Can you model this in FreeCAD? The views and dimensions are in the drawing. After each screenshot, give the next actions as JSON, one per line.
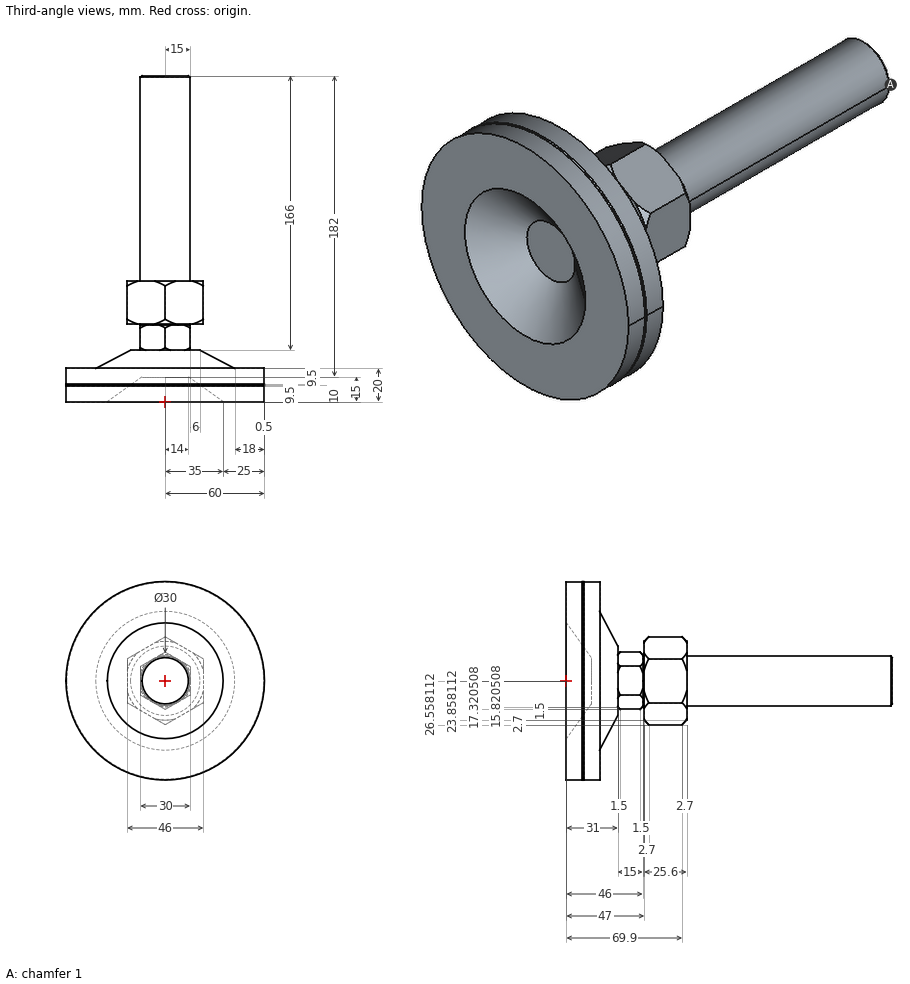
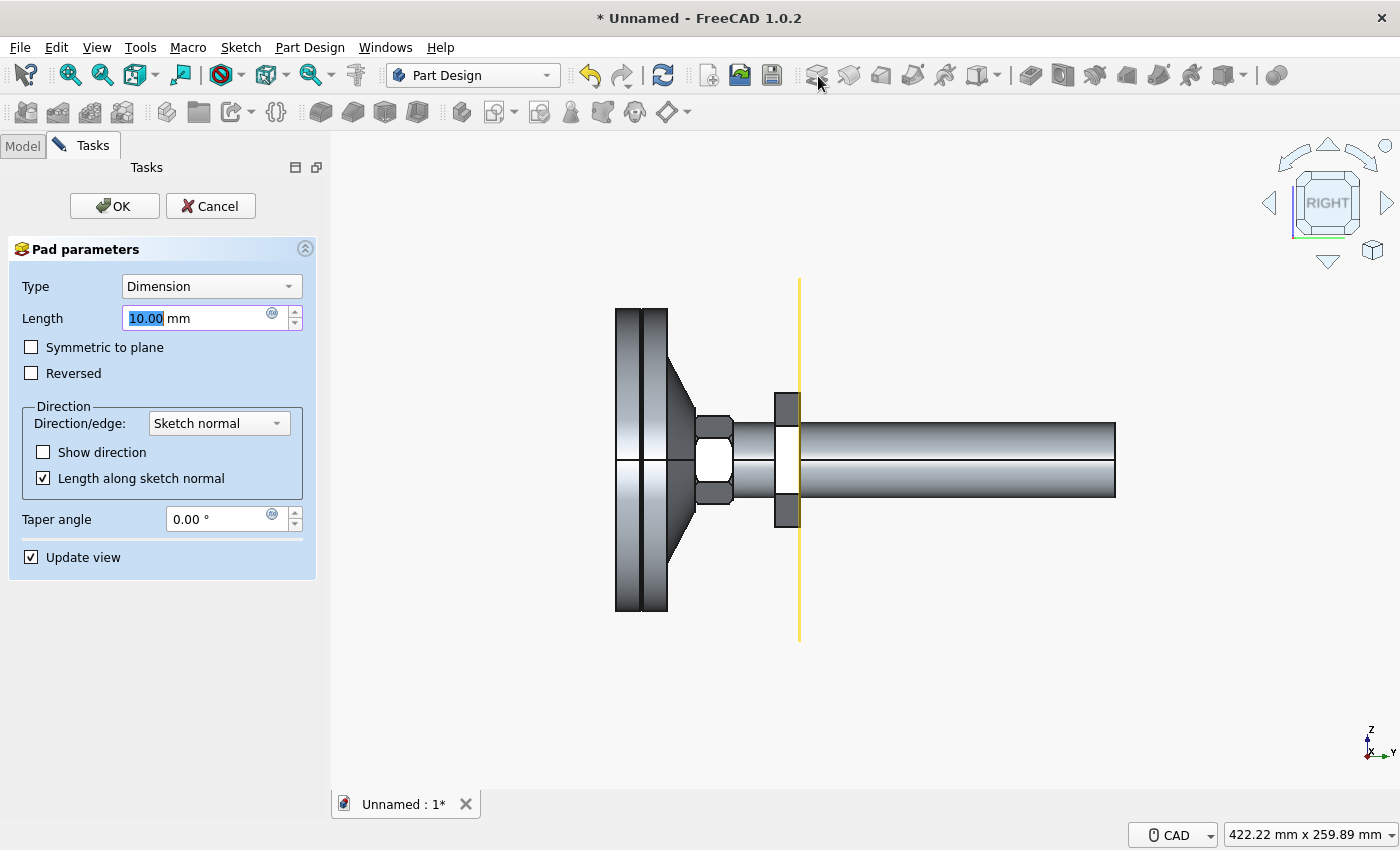
{"action": "type", "text": "25.6"}
{"action": "key", "text": "Tab"}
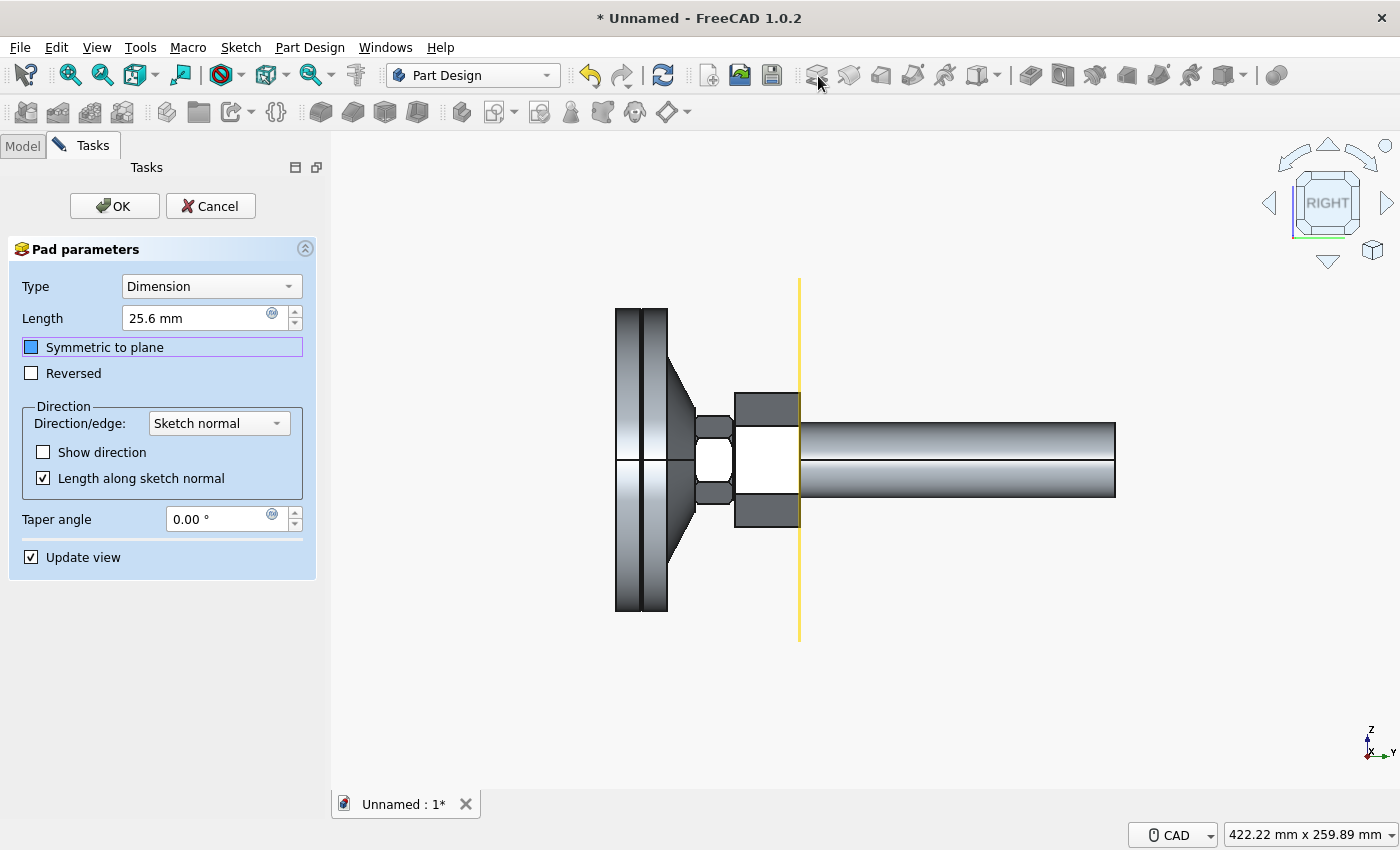
{"action": "left_click", "coordinate": [115, 206]}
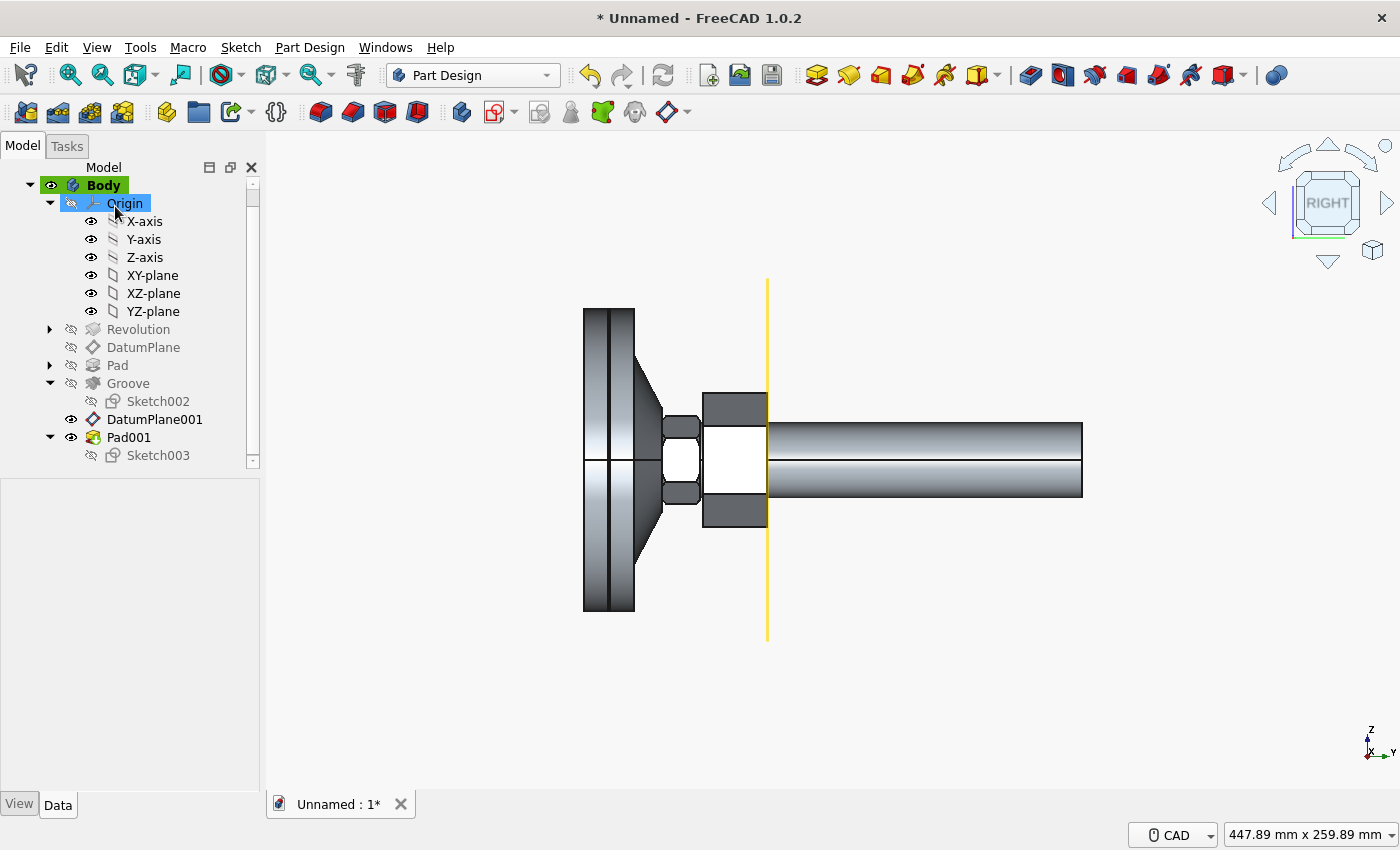
{"action": "left_click", "coordinate": [116, 419]}
{"action": "key", "text": "space"}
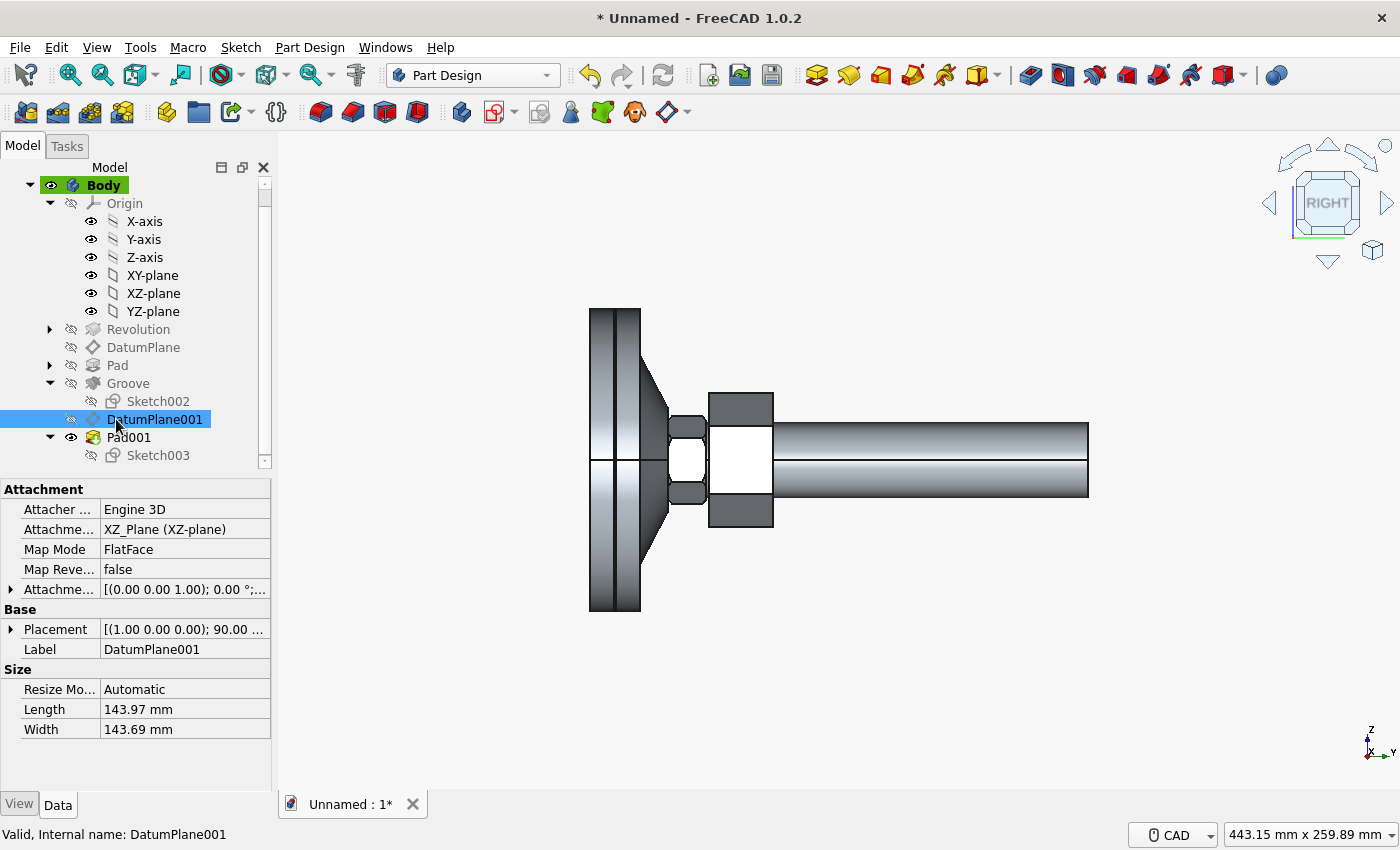
{"action": "left_click", "coordinate": [318, 749]}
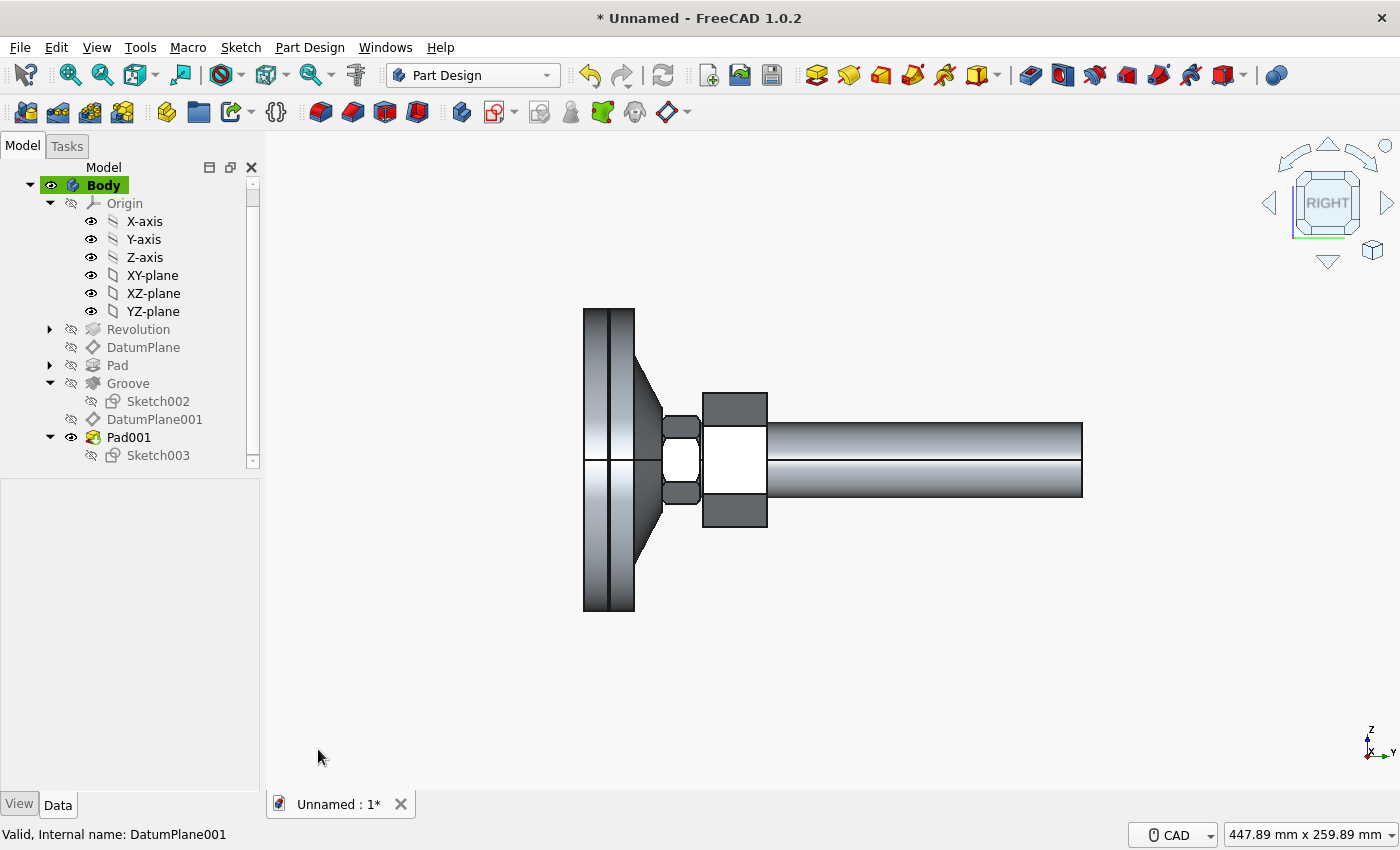
{"action": "left_click", "coordinate": [494, 112]}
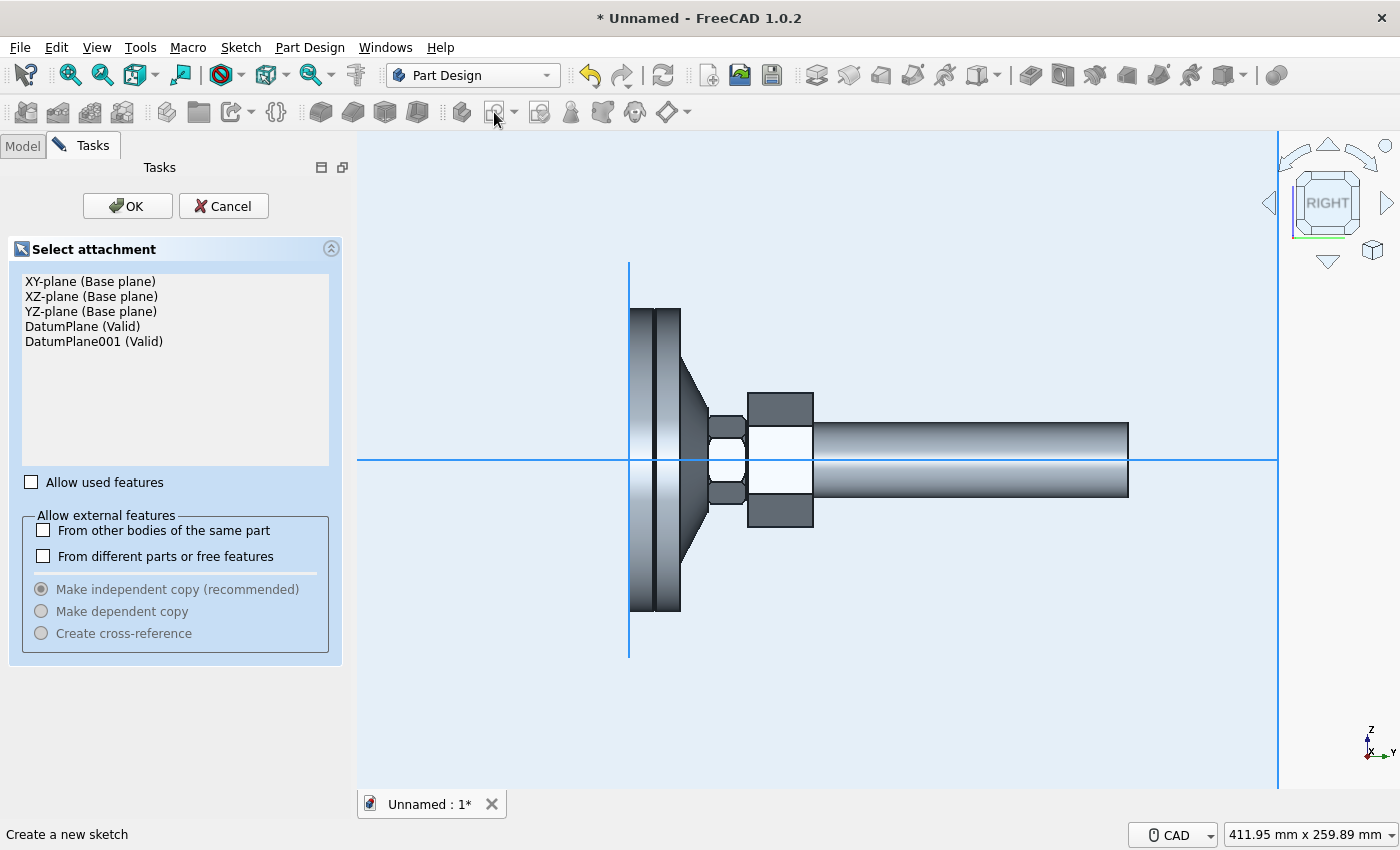
{"action": "left_click", "coordinate": [82, 312]}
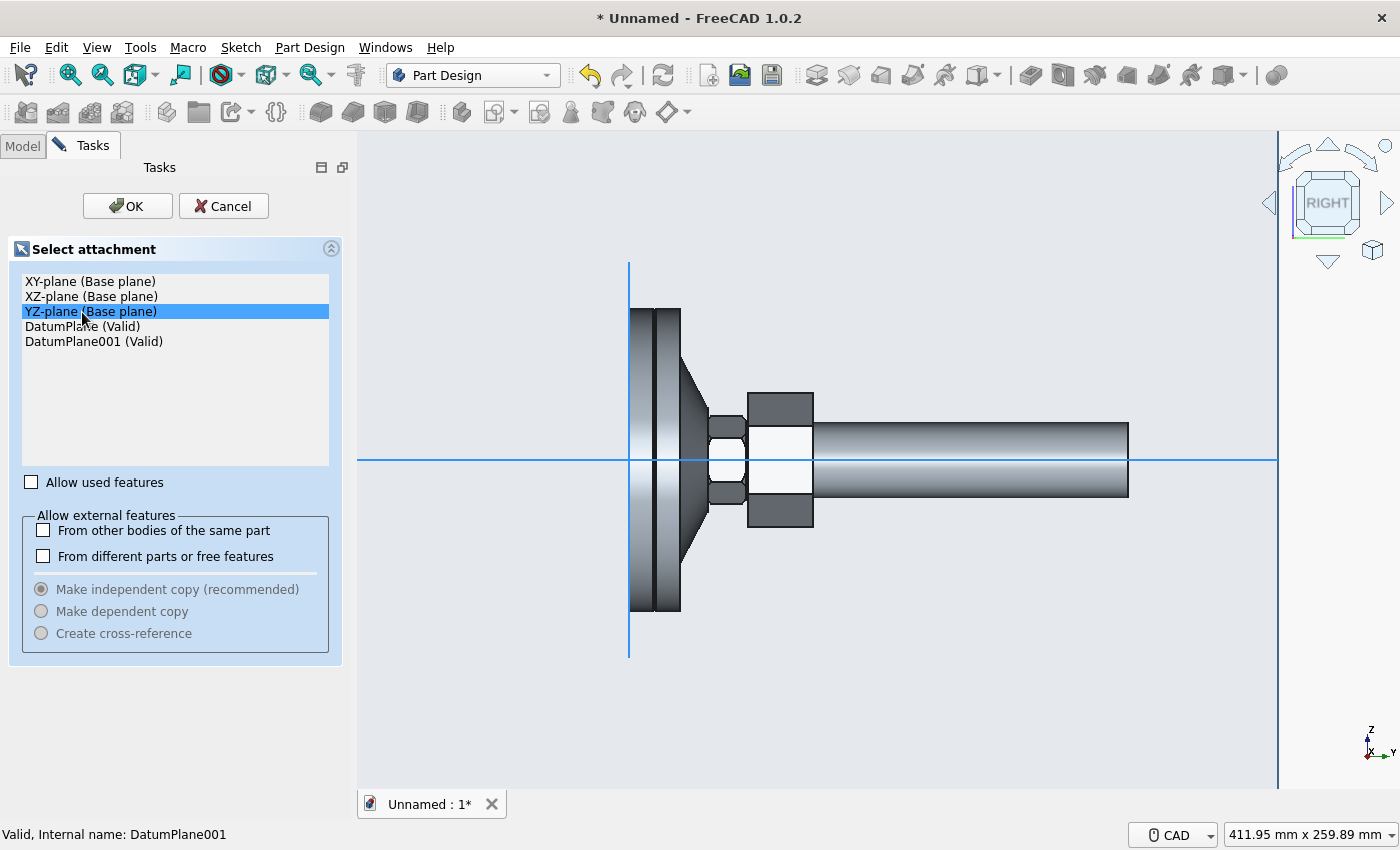
{"action": "left_click", "coordinate": [128, 206]}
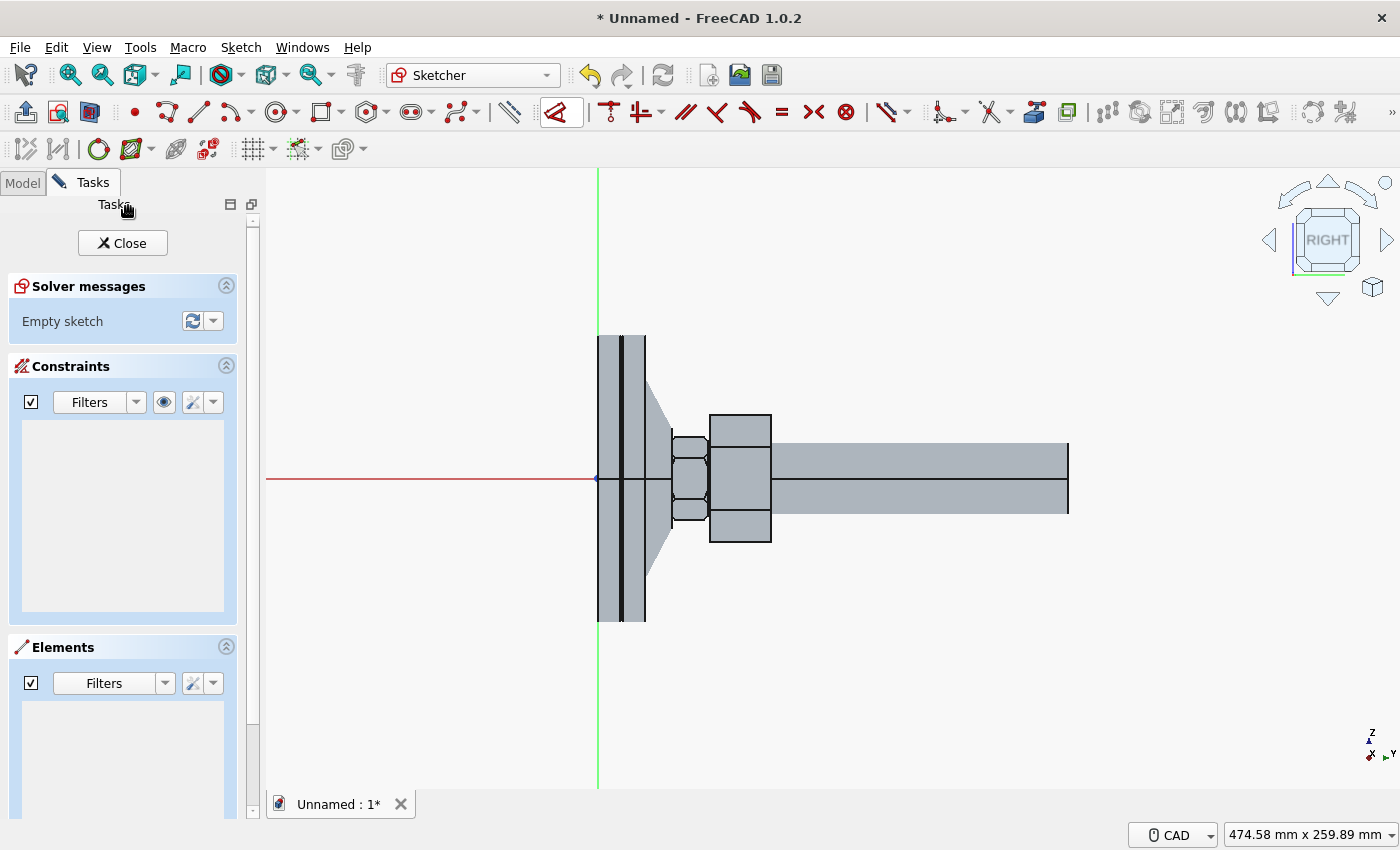
{"action": "key", "text": "q s"}